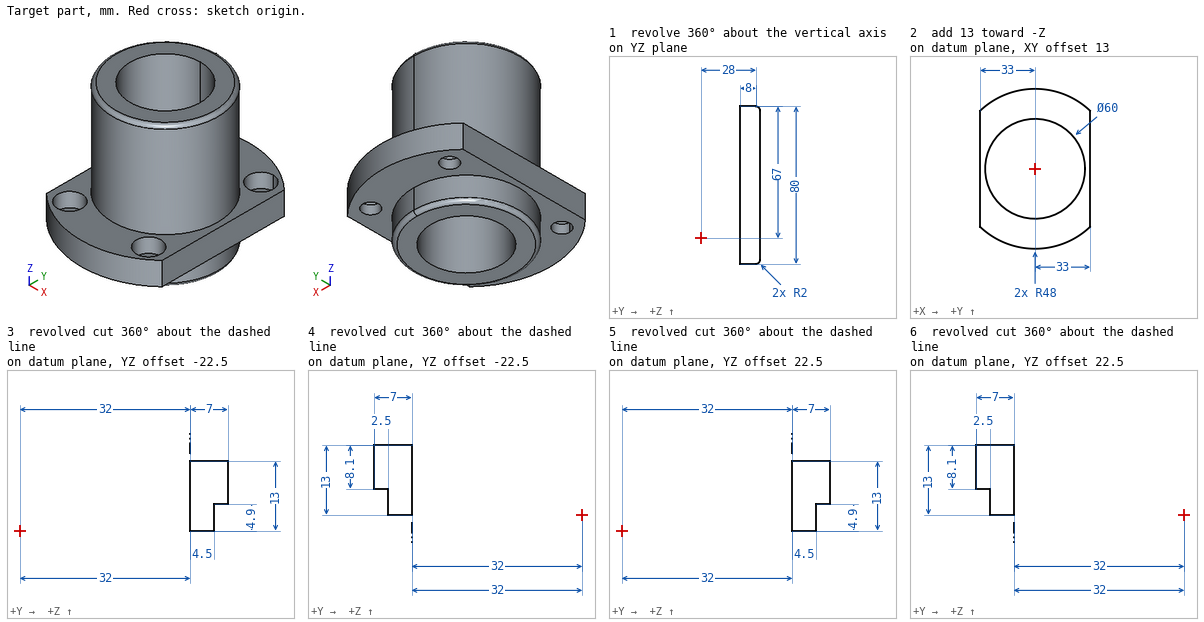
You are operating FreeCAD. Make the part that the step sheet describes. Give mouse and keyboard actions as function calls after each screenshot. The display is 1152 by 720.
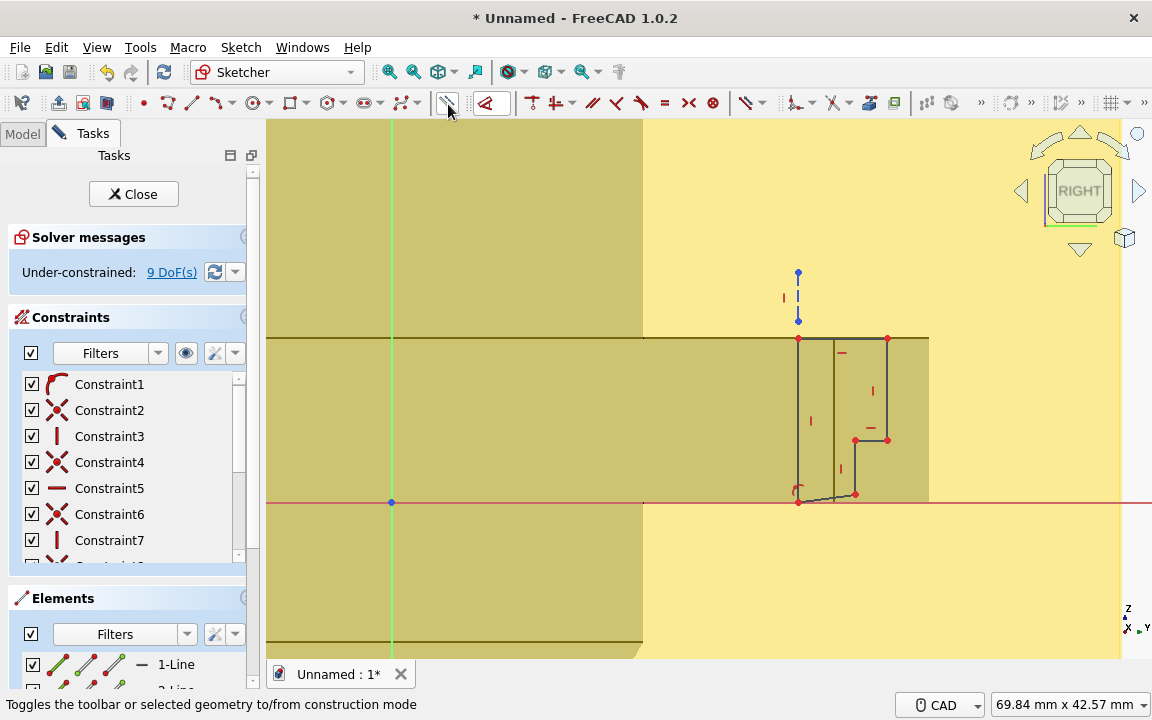
click(815, 500)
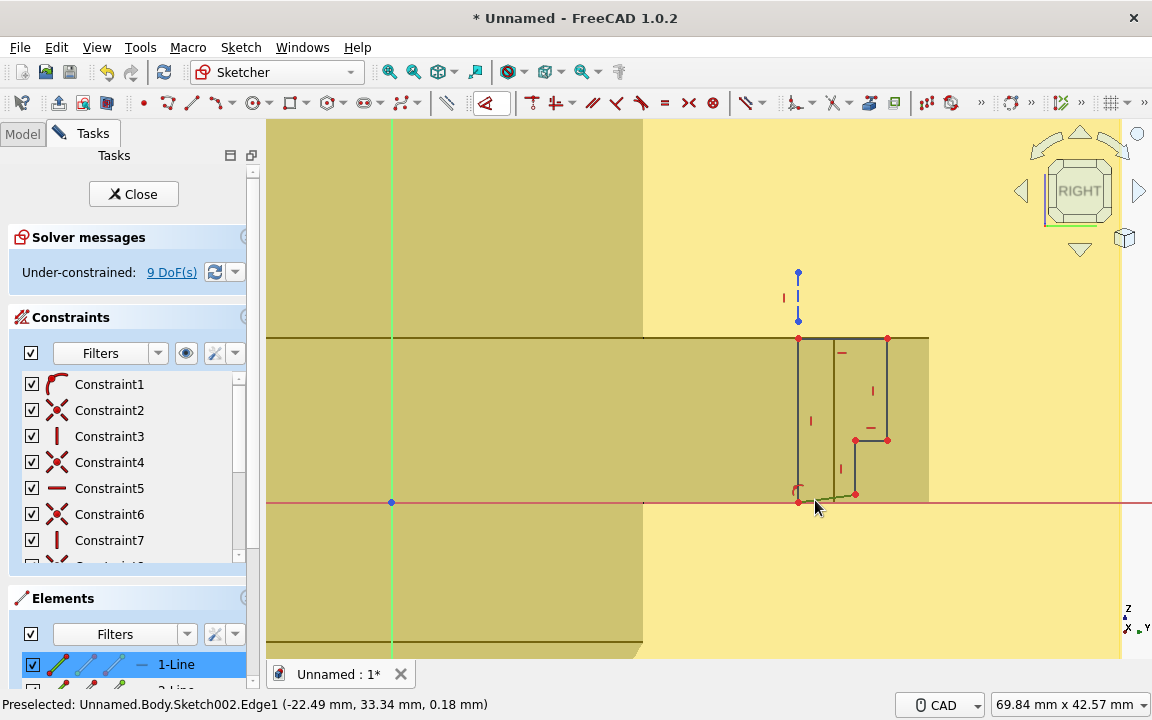
click(574, 104)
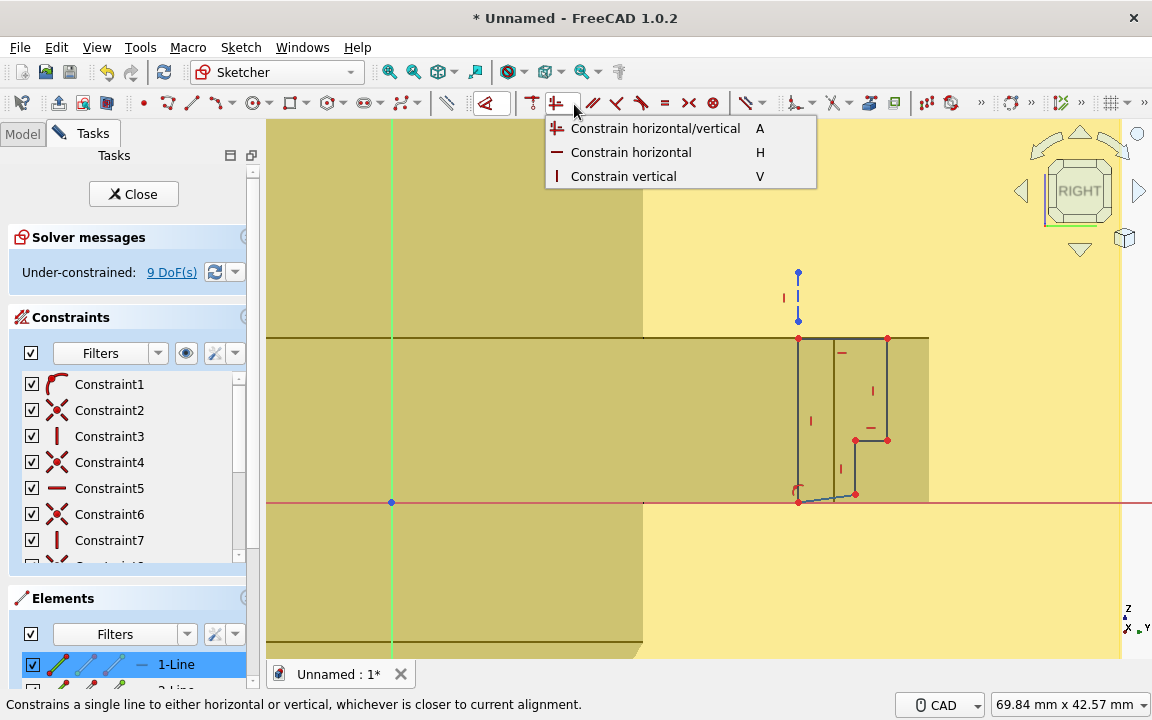
click(681, 152)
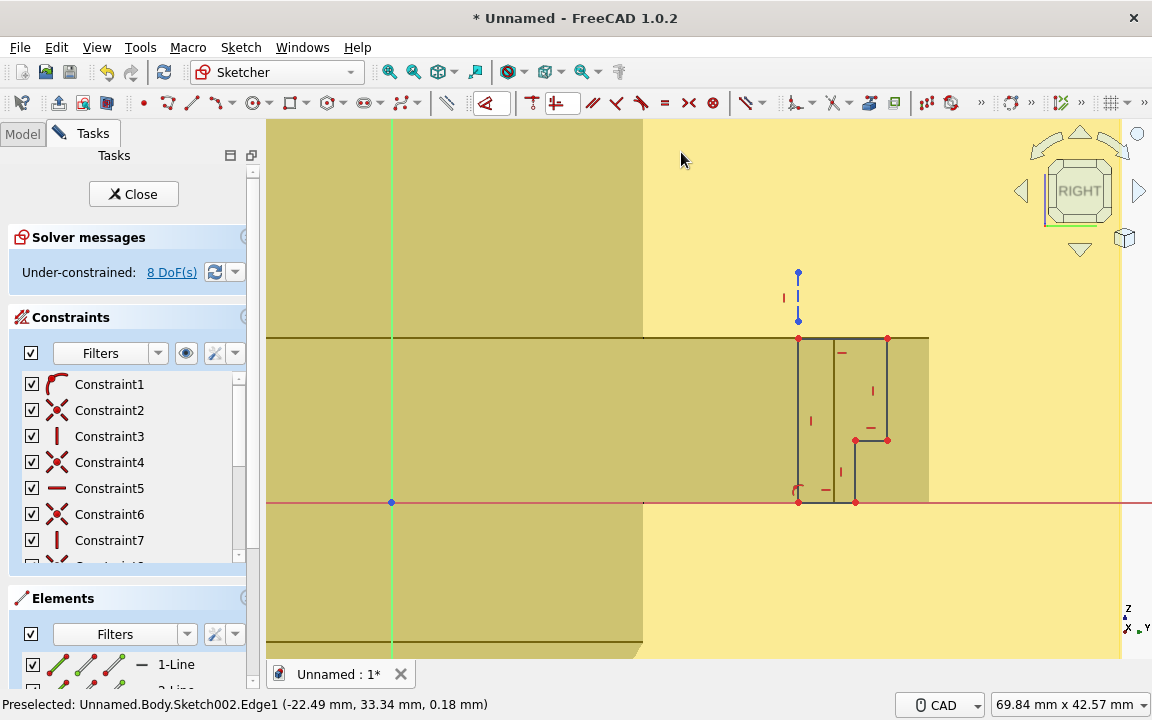
click(860, 339)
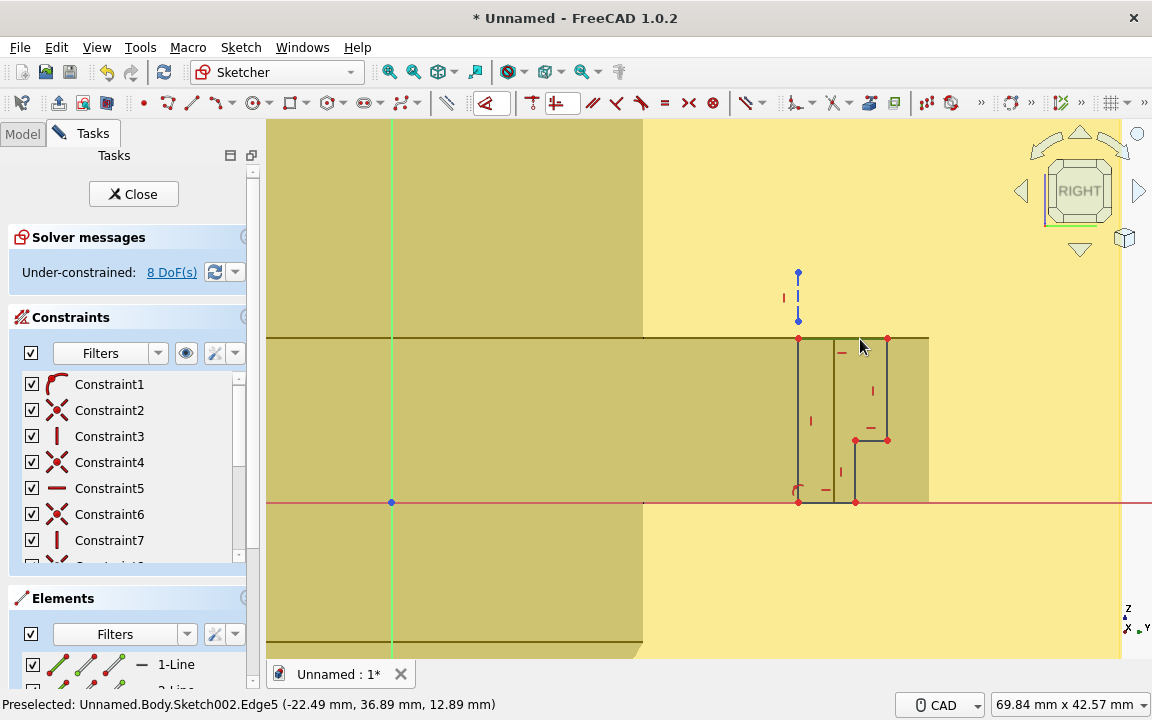
key(l)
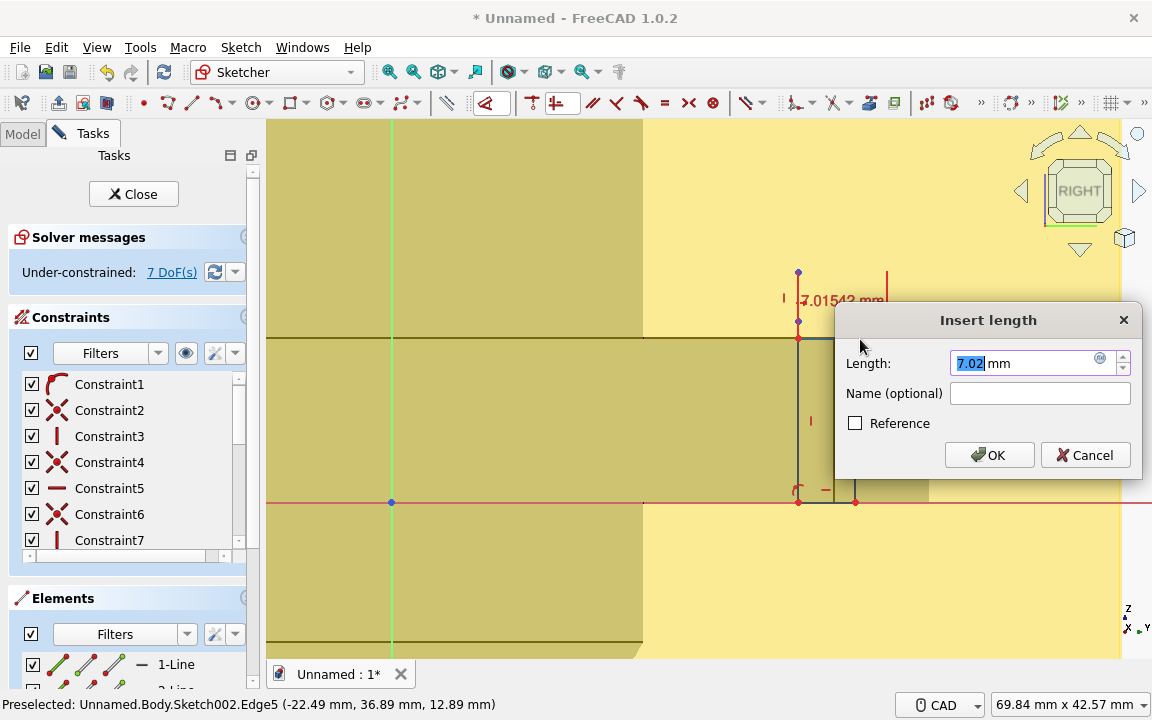
text(7)
key(Return)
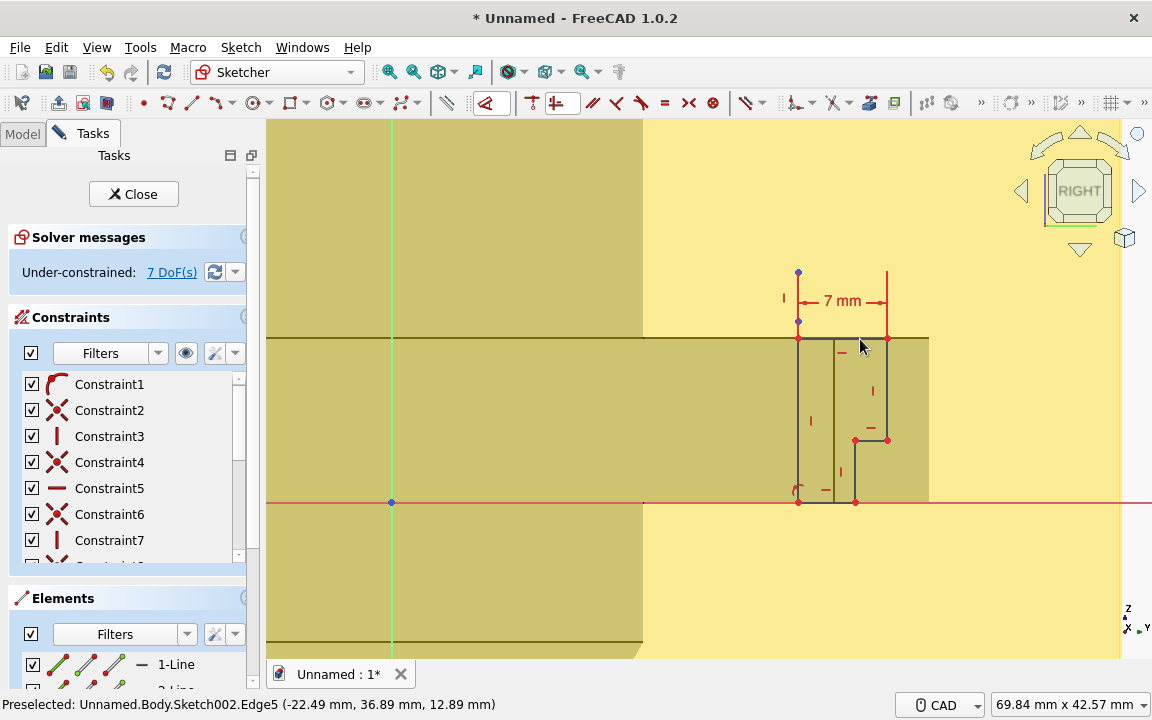
click(798, 388)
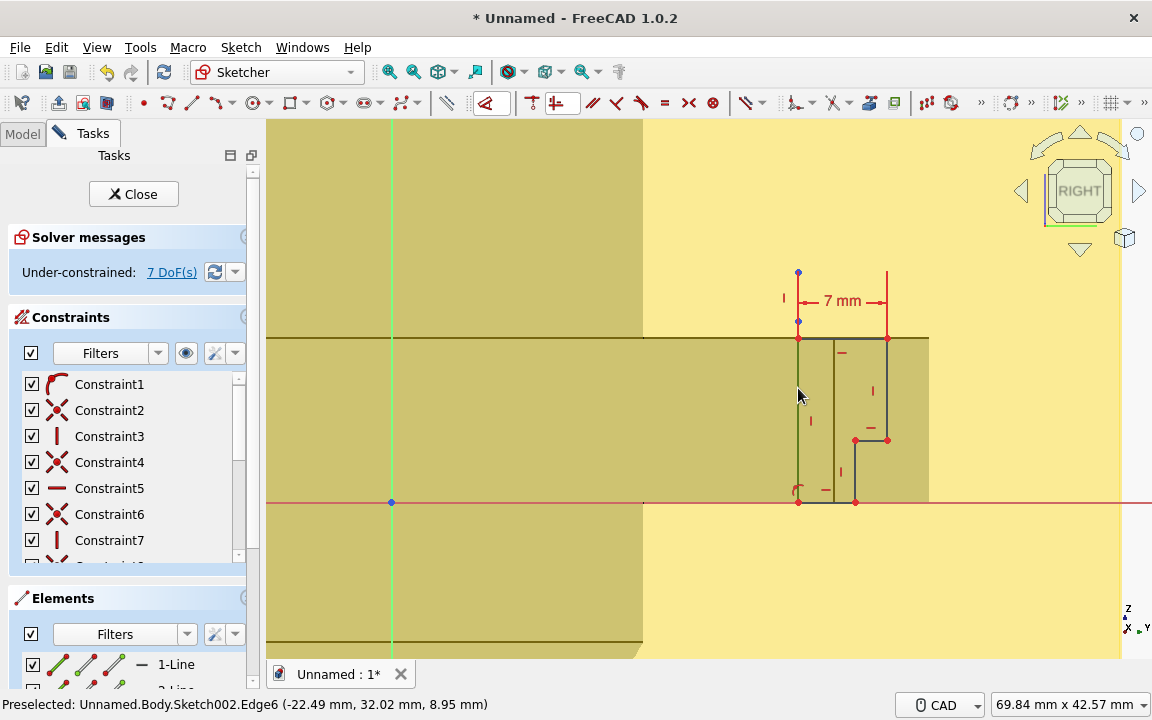
key(i)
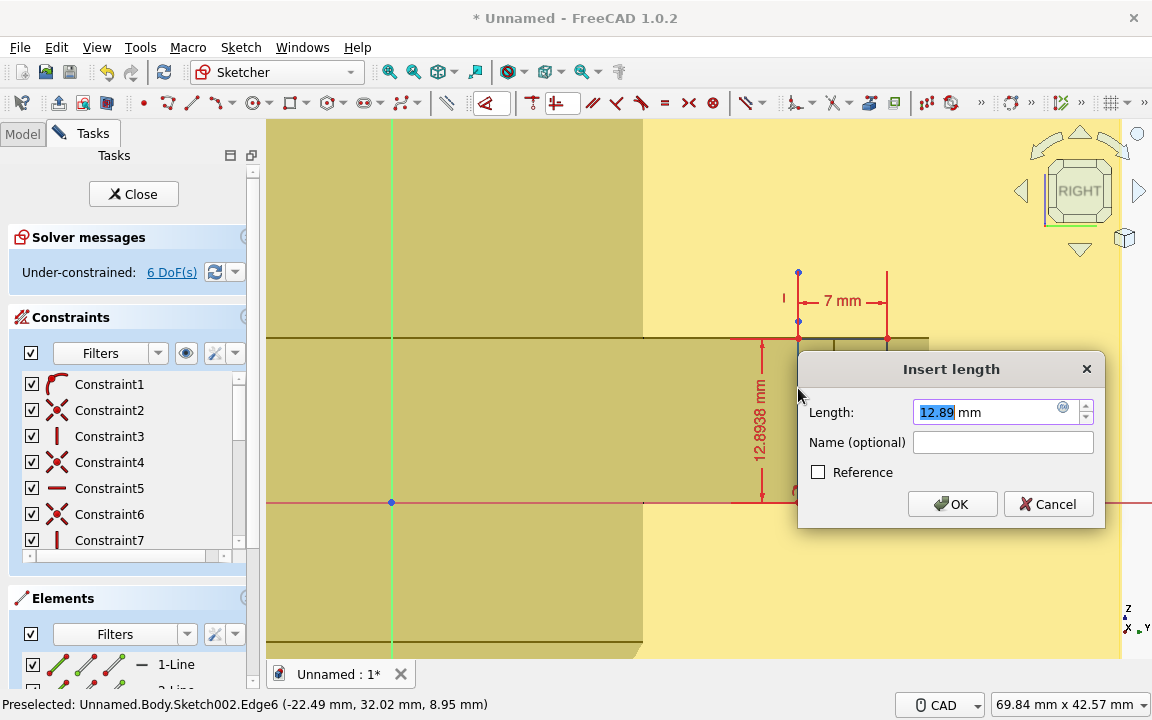
text(13)
key(Return)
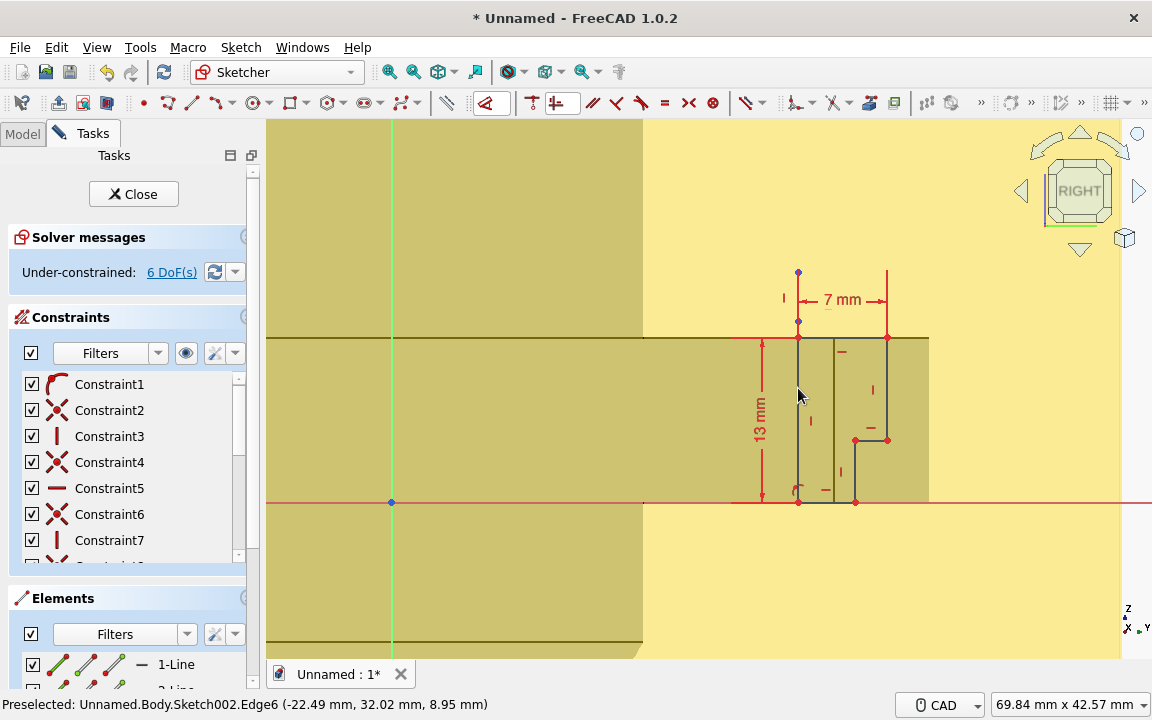
click(815, 503)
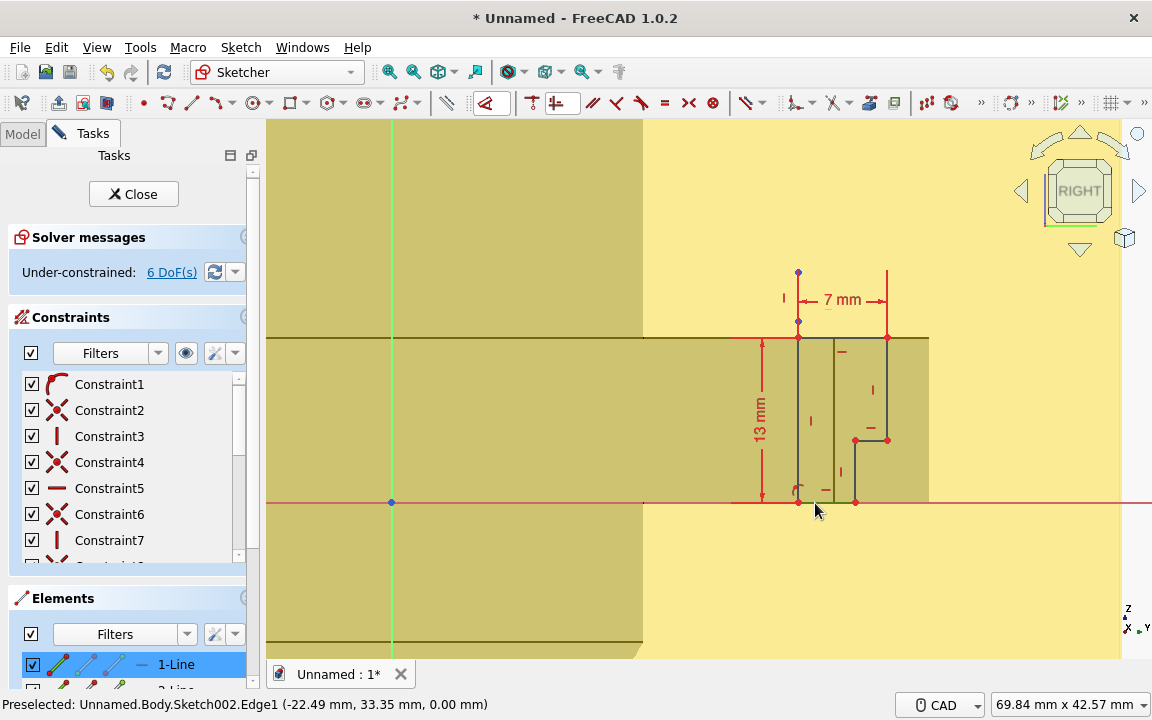
click(504, 104)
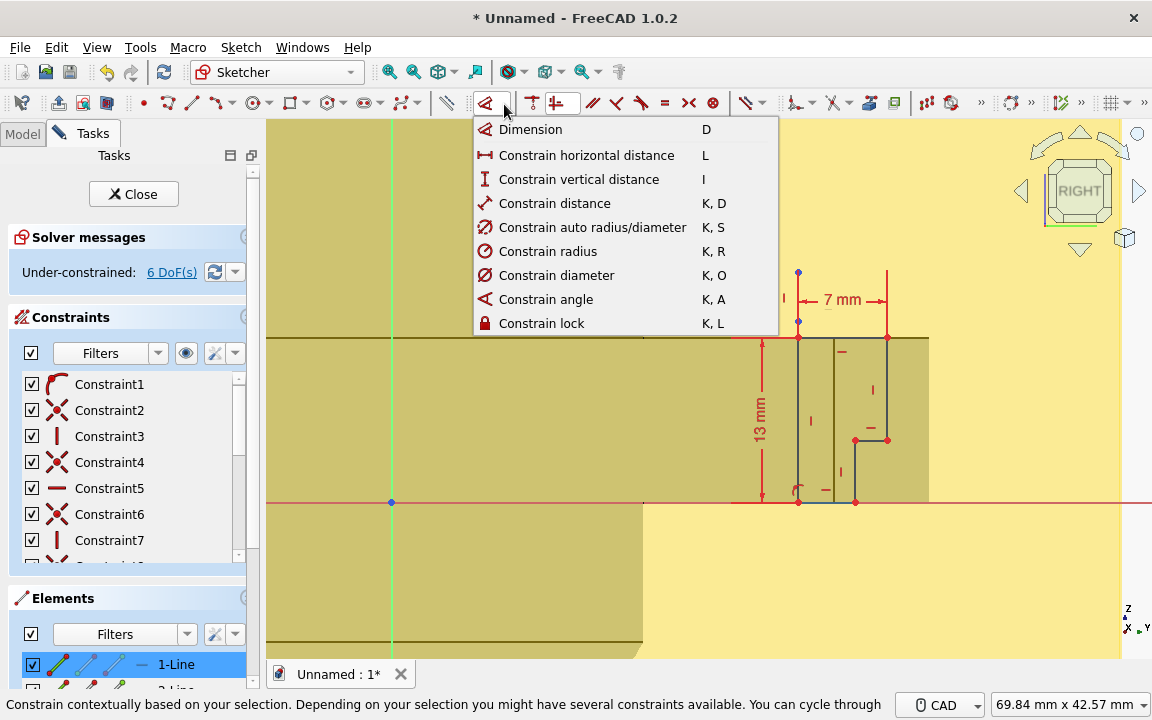
click(626, 155)